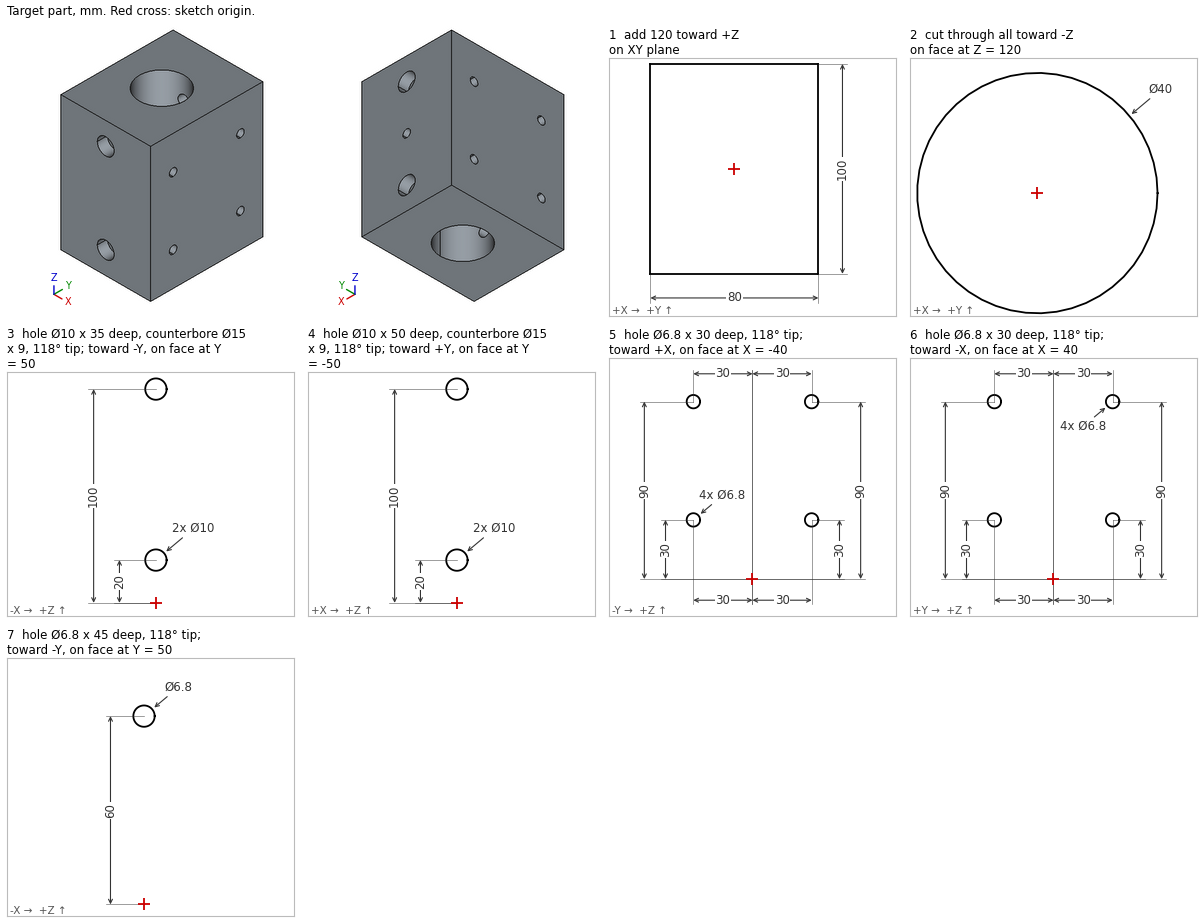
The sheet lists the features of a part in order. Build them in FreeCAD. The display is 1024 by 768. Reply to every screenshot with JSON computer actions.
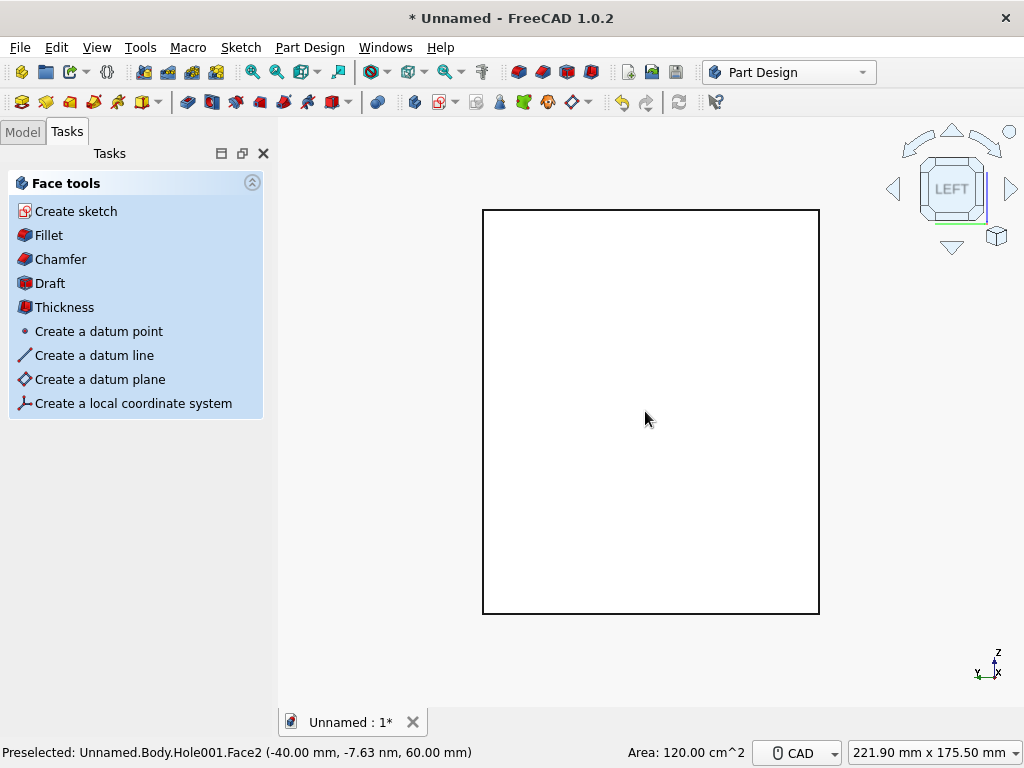
{"action": "left_click", "coordinate": [440, 102]}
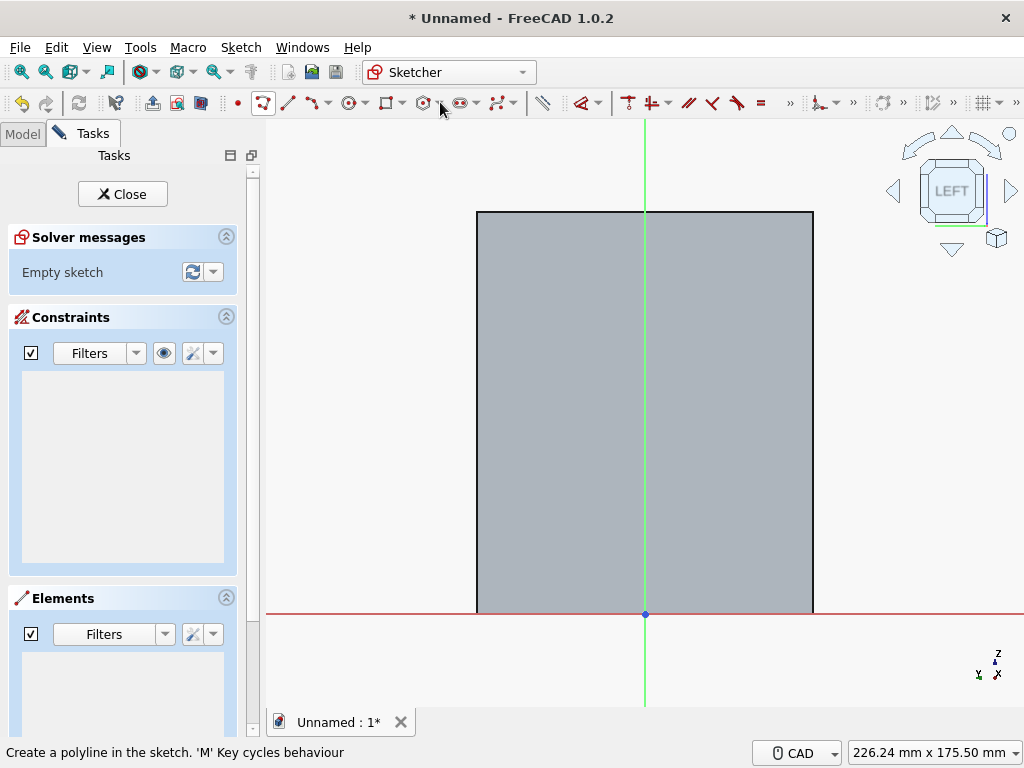
{"action": "left_click", "coordinate": [350, 104]}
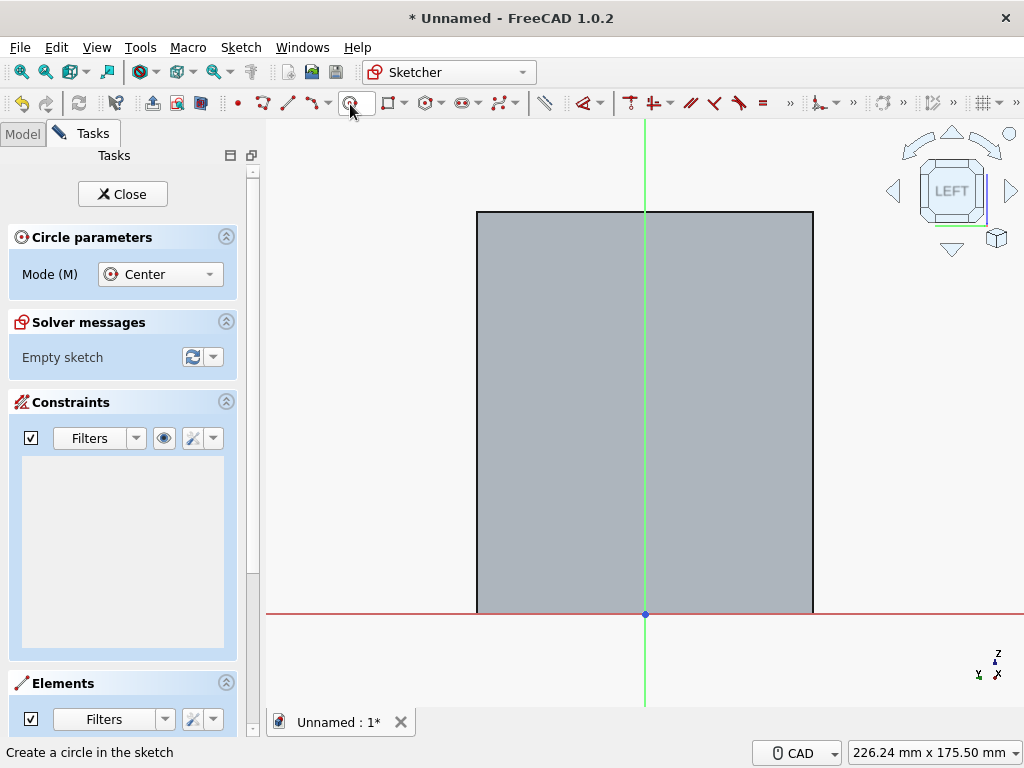
{"action": "scroll", "coordinate": [544, 514], "scroll_direction": "up", "scroll_amount": 4}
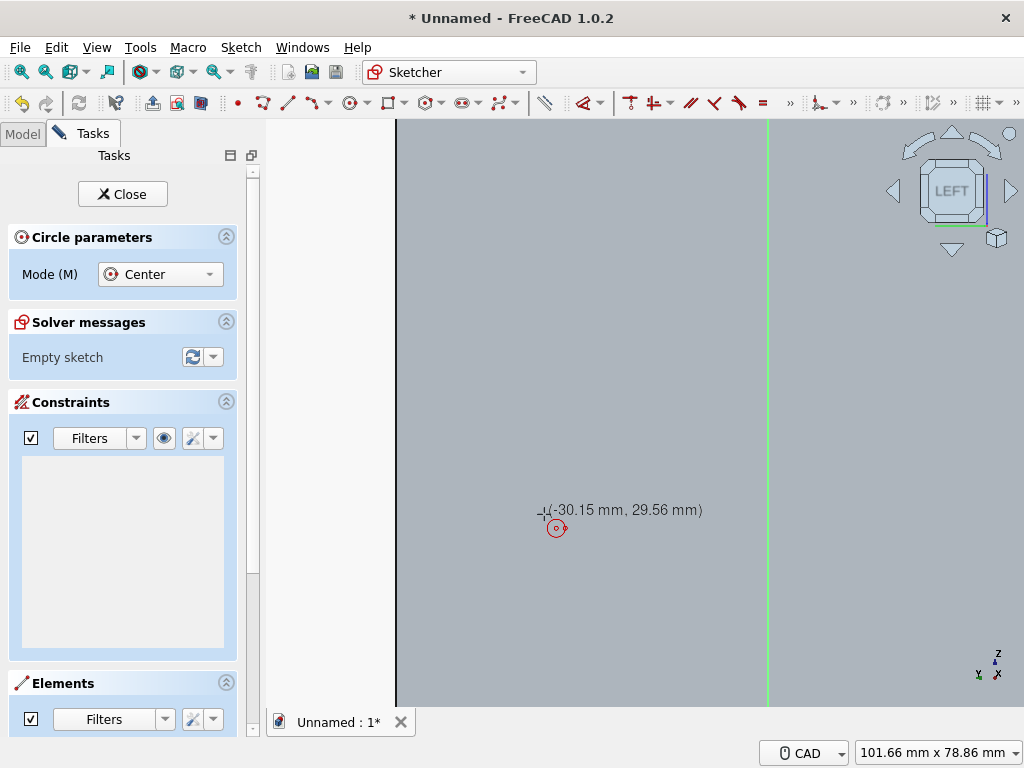
{"action": "left_click", "coordinate": [545, 512]}
{"action": "mouse_move", "coordinate": [563, 494]}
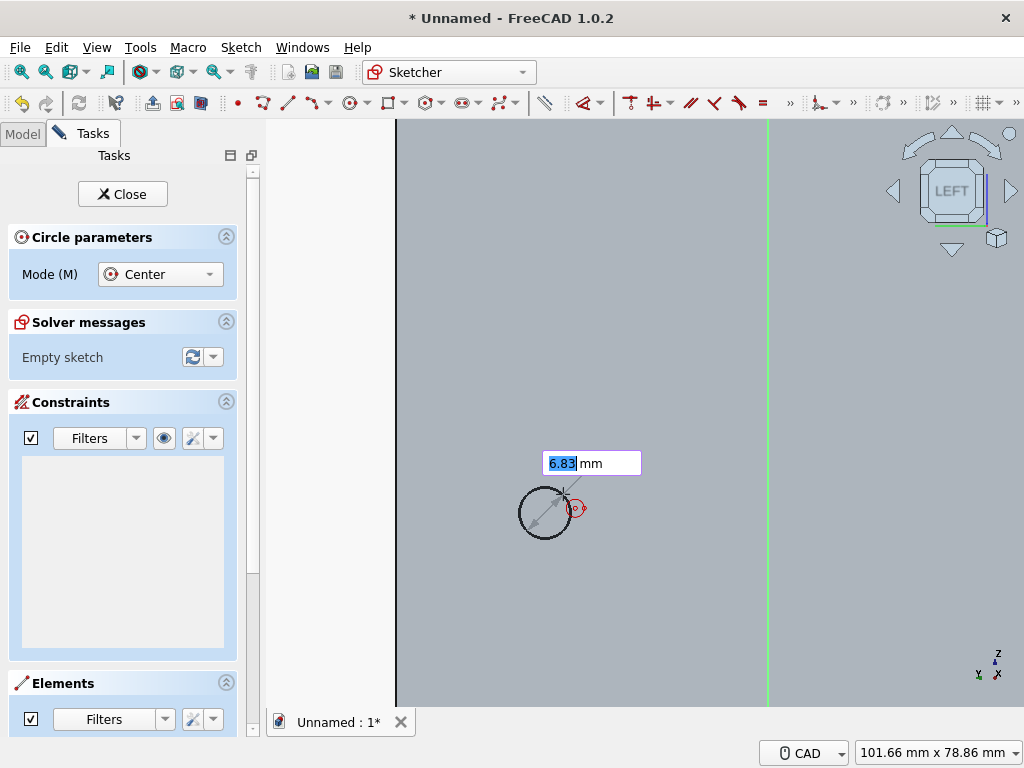
{"action": "type", "text": "6.8"}
{"action": "key", "text": "Return"}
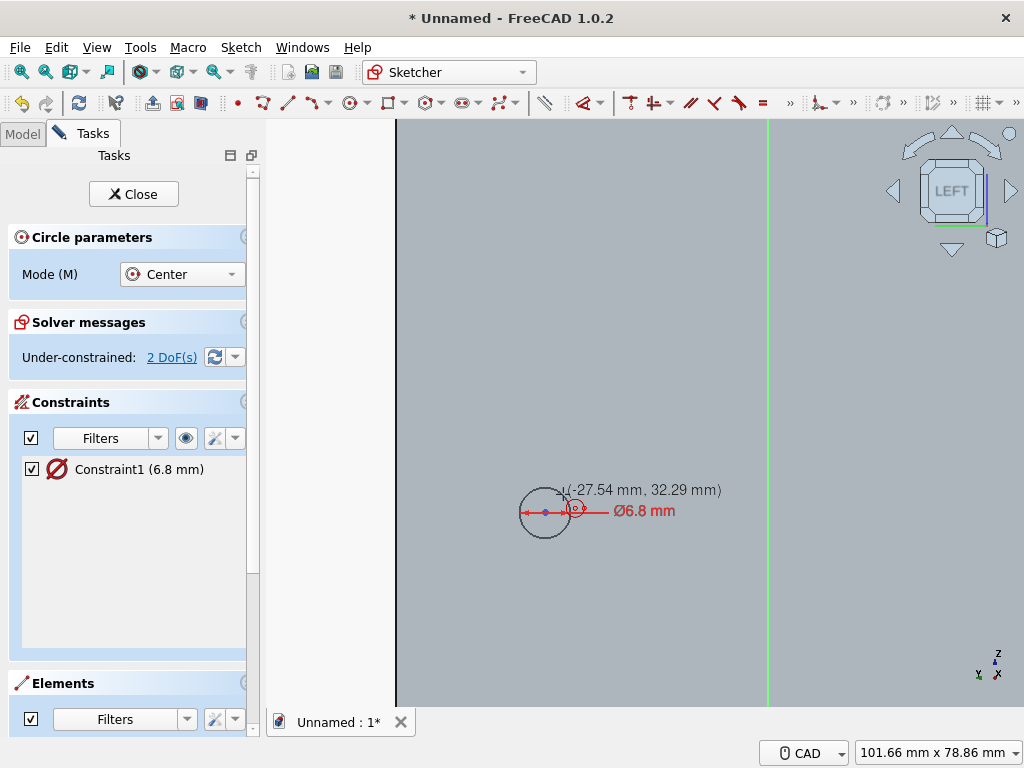
{"action": "scroll", "coordinate": [343, 444], "scroll_direction": "down", "scroll_amount": 3}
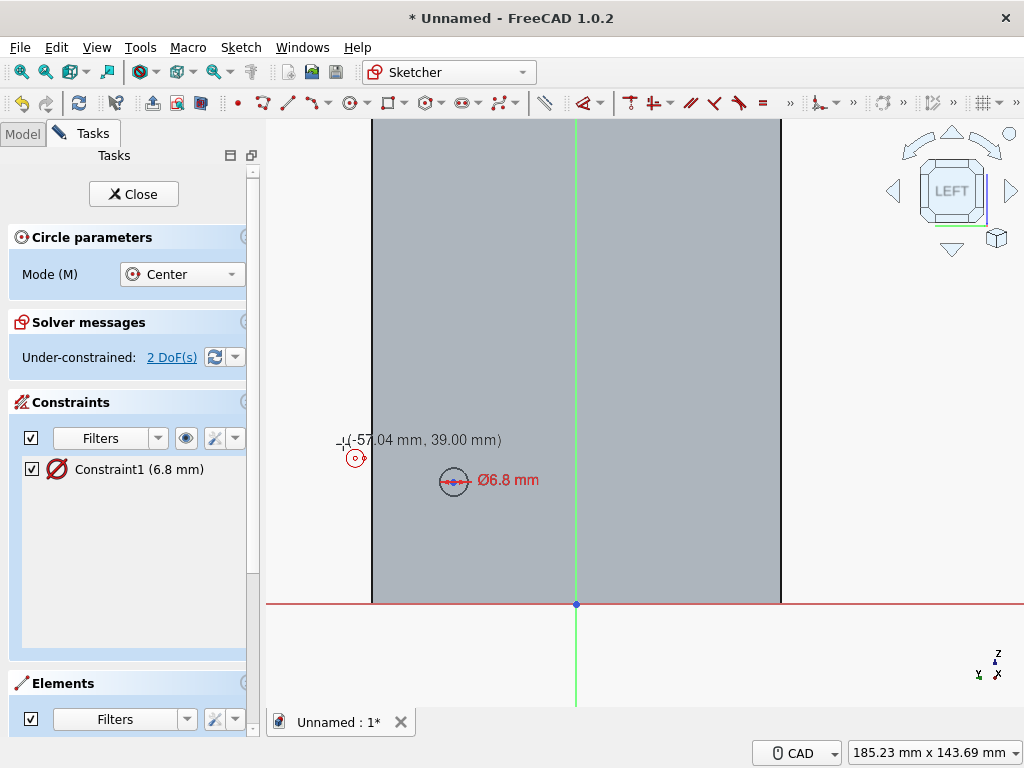
{"action": "scroll", "coordinate": [454, 236], "scroll_direction": "up", "scroll_amount": 3}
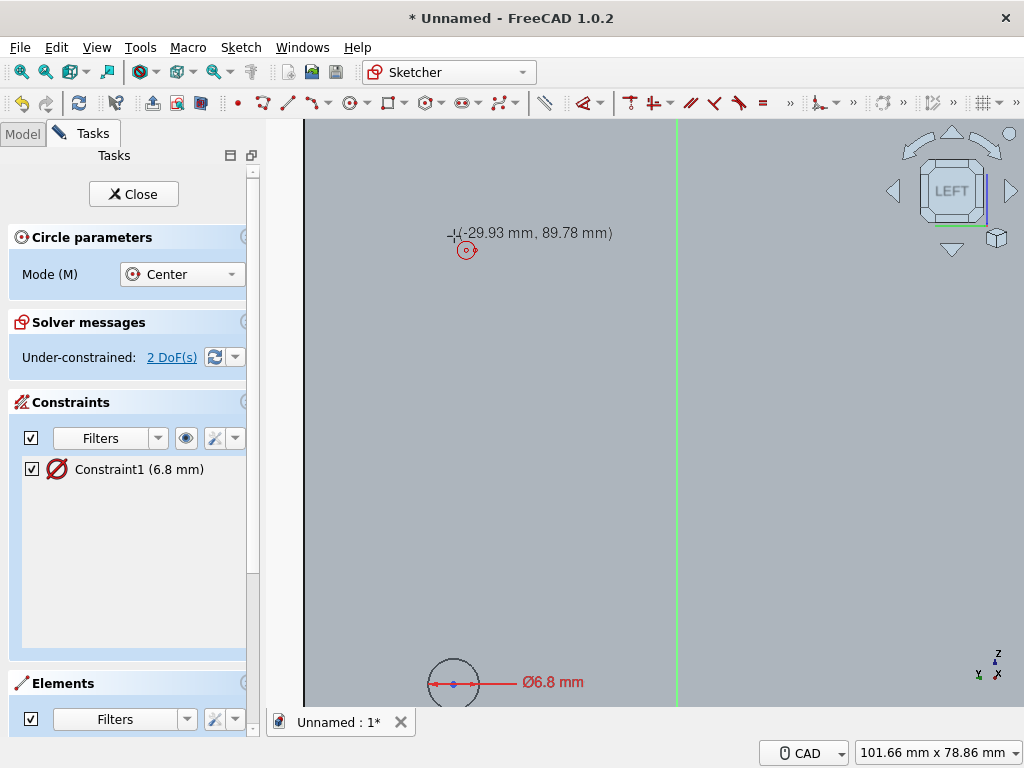
{"action": "left_click", "coordinate": [453, 236]}
{"action": "mouse_move", "coordinate": [471, 218]}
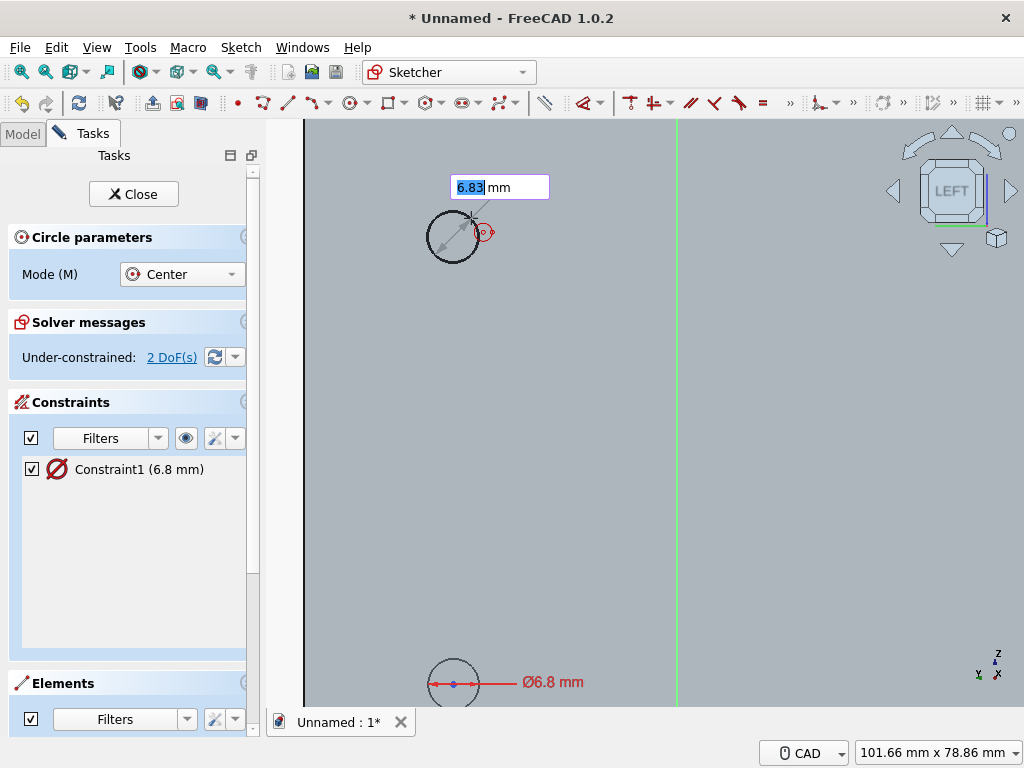
{"action": "type", "text": "6.8"}
{"action": "key", "text": "Return"}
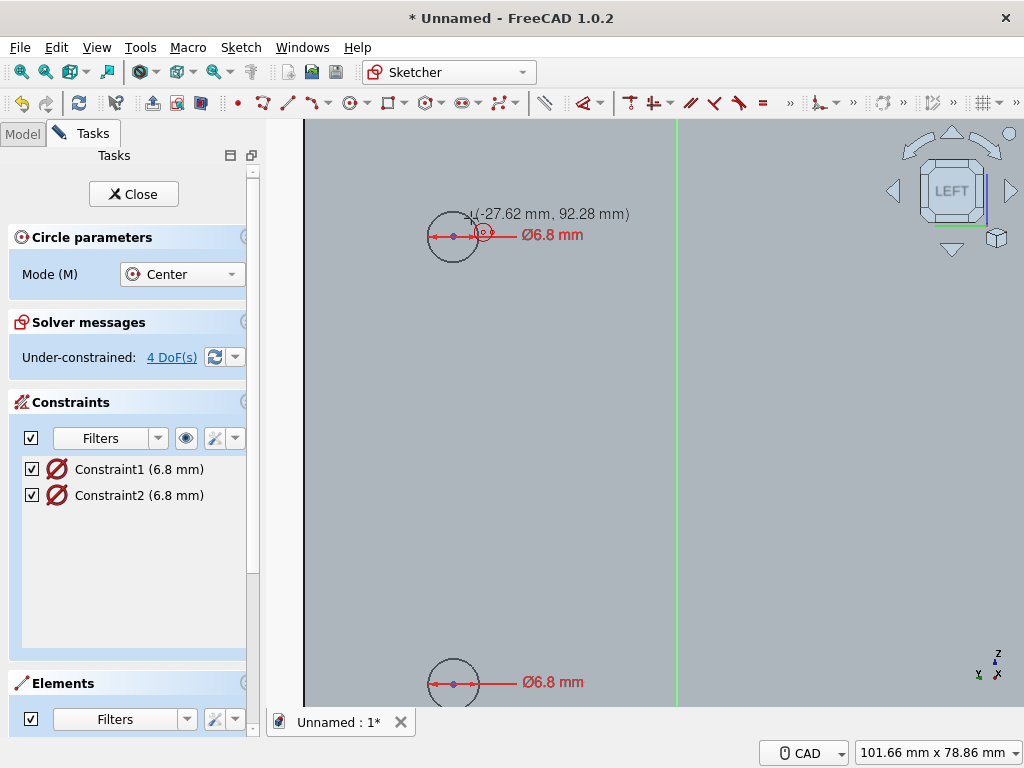
{"action": "scroll", "coordinate": [454, 236], "scroll_direction": "down", "scroll_amount": 3}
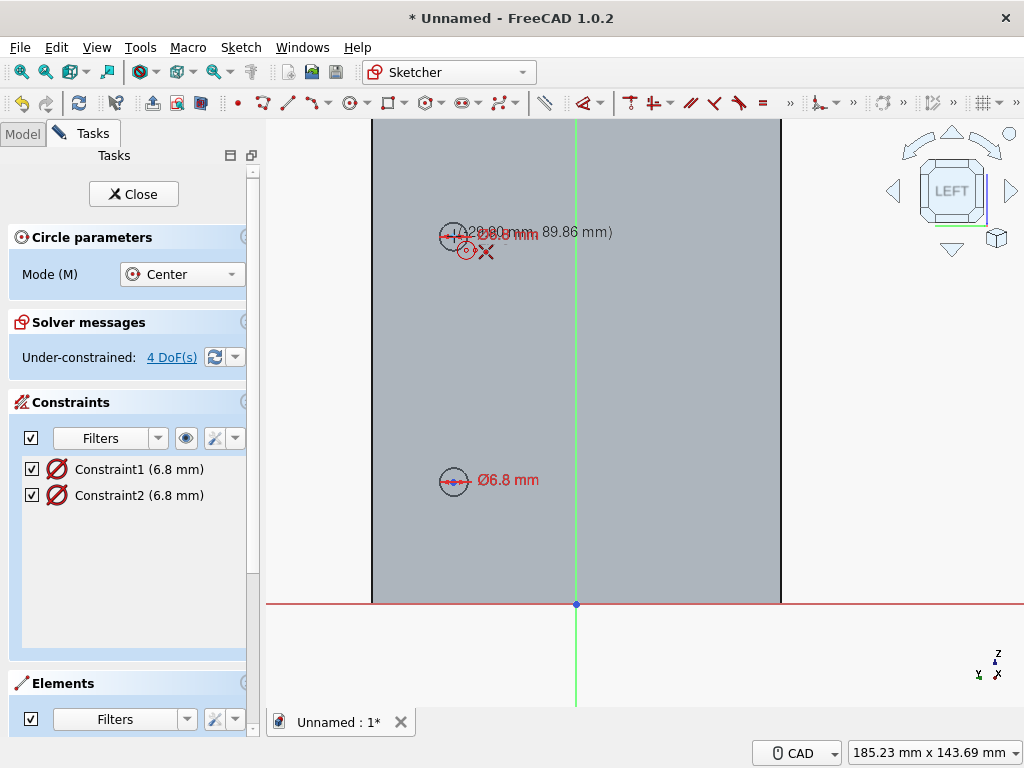
{"action": "scroll", "coordinate": [699, 236], "scroll_direction": "up", "scroll_amount": 3}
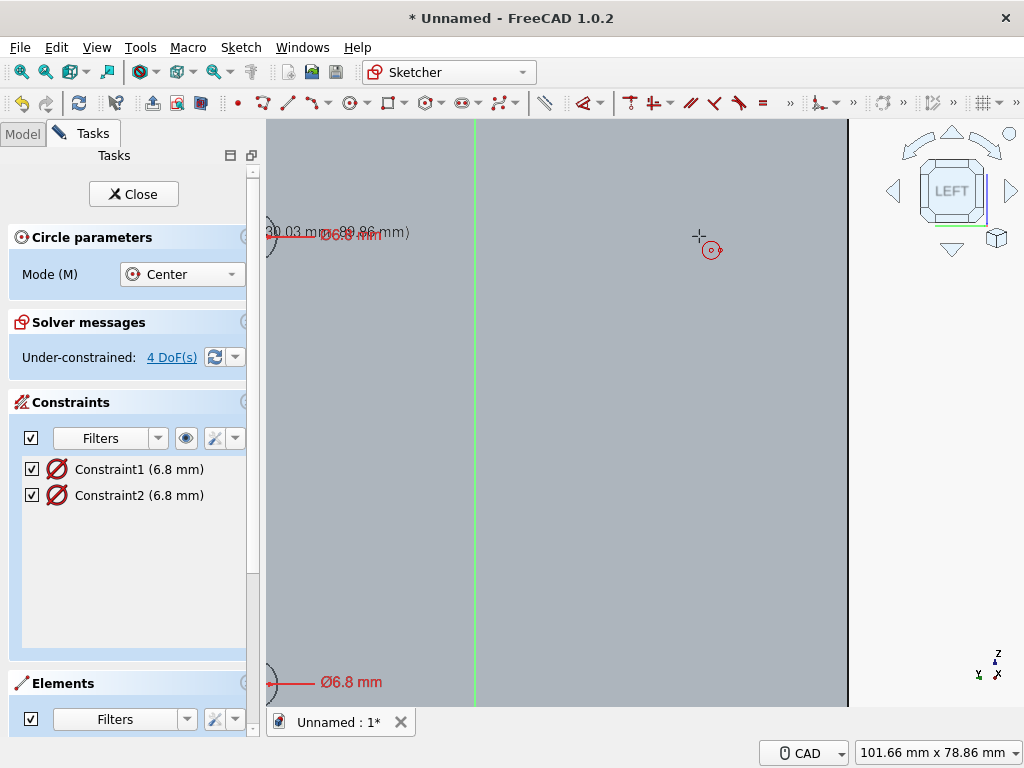
{"action": "left_click", "coordinate": [699, 236]}
{"action": "mouse_move", "coordinate": [717, 218]}